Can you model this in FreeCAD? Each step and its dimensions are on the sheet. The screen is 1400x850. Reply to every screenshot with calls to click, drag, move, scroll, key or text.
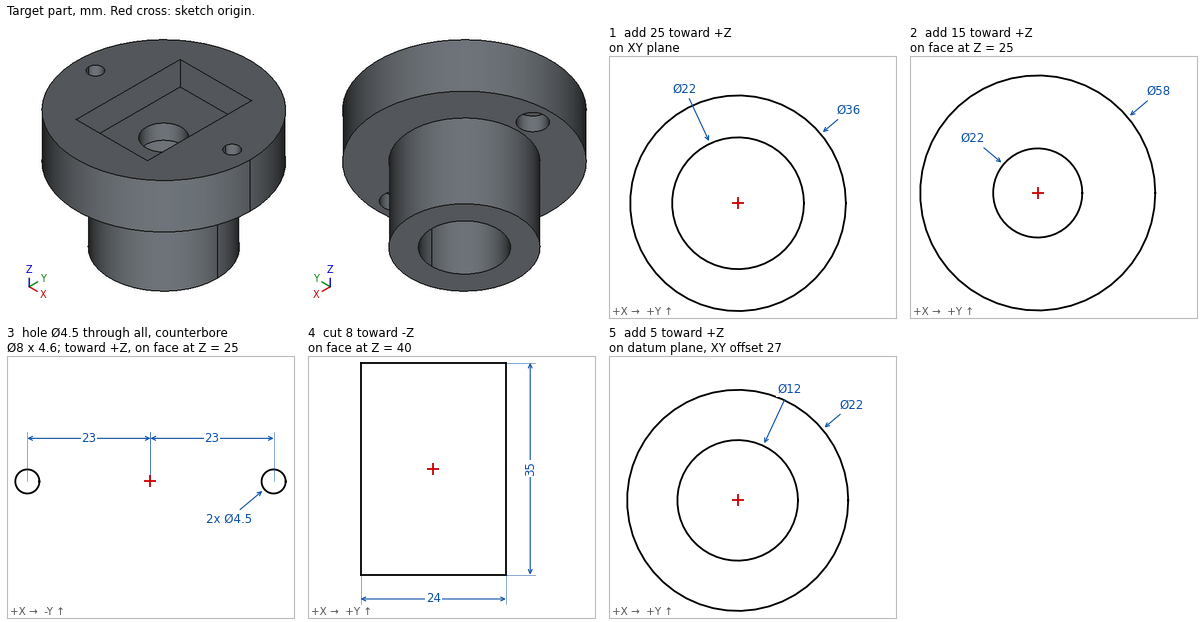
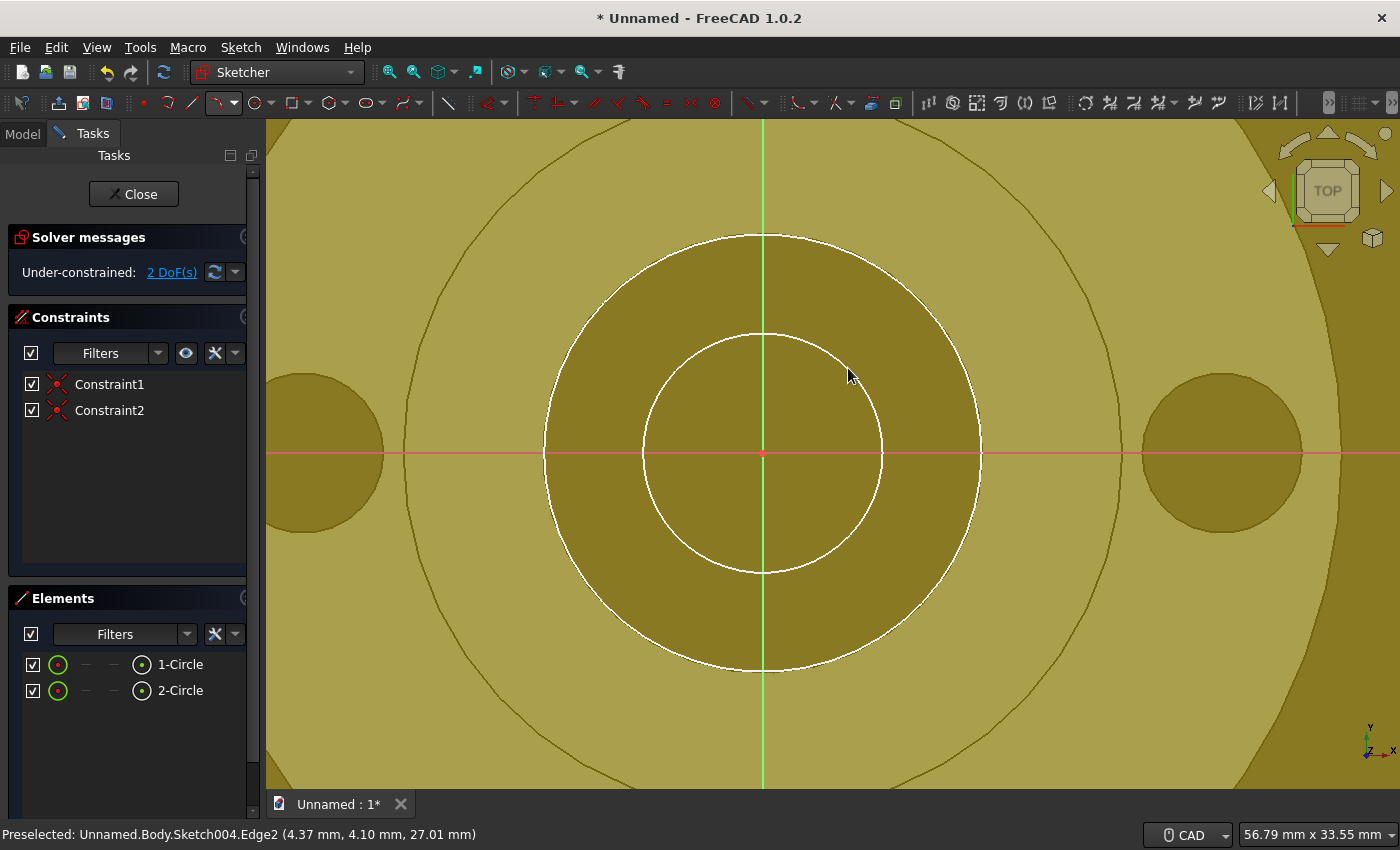
key(d)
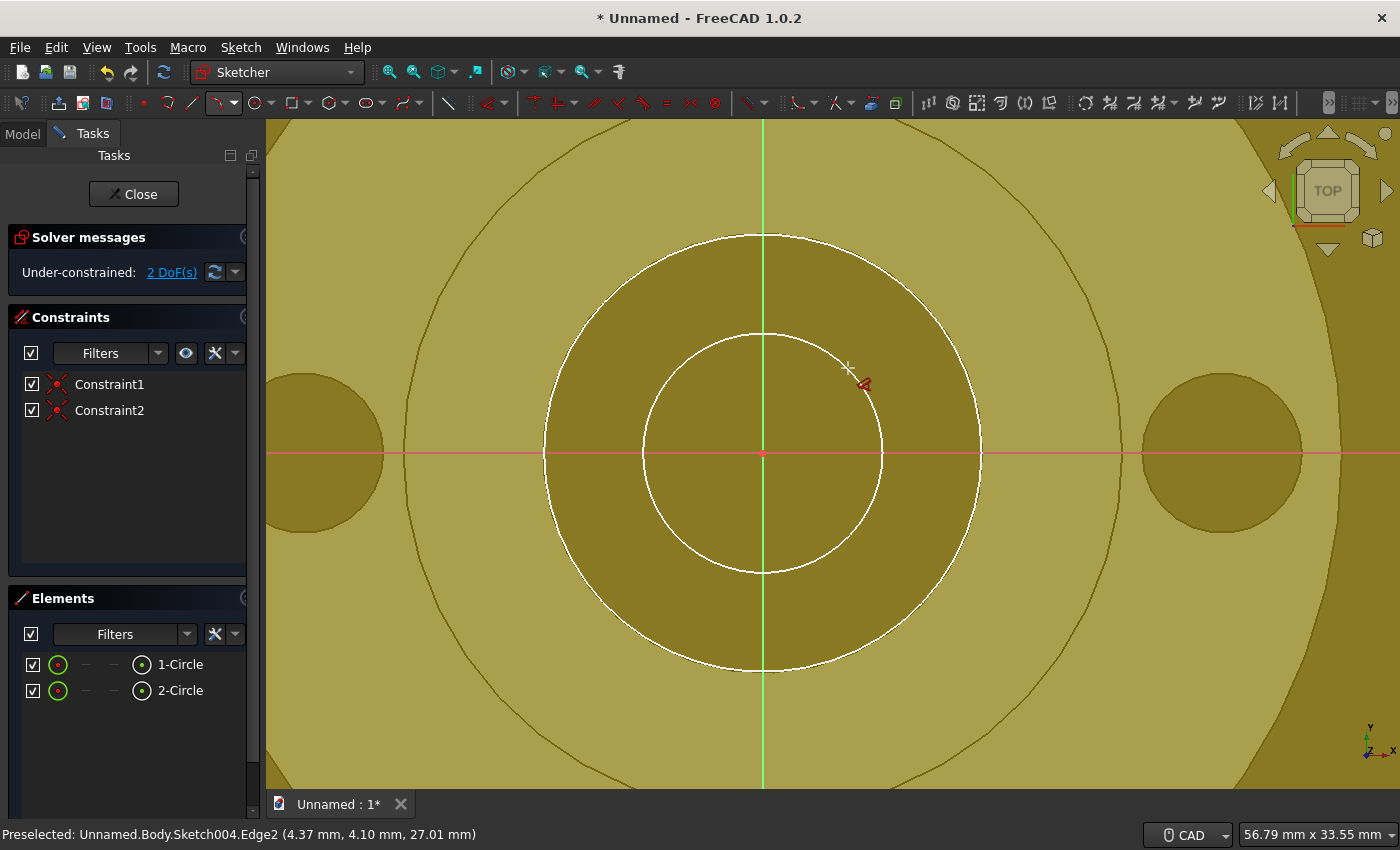
click(917, 298)
click(940, 275)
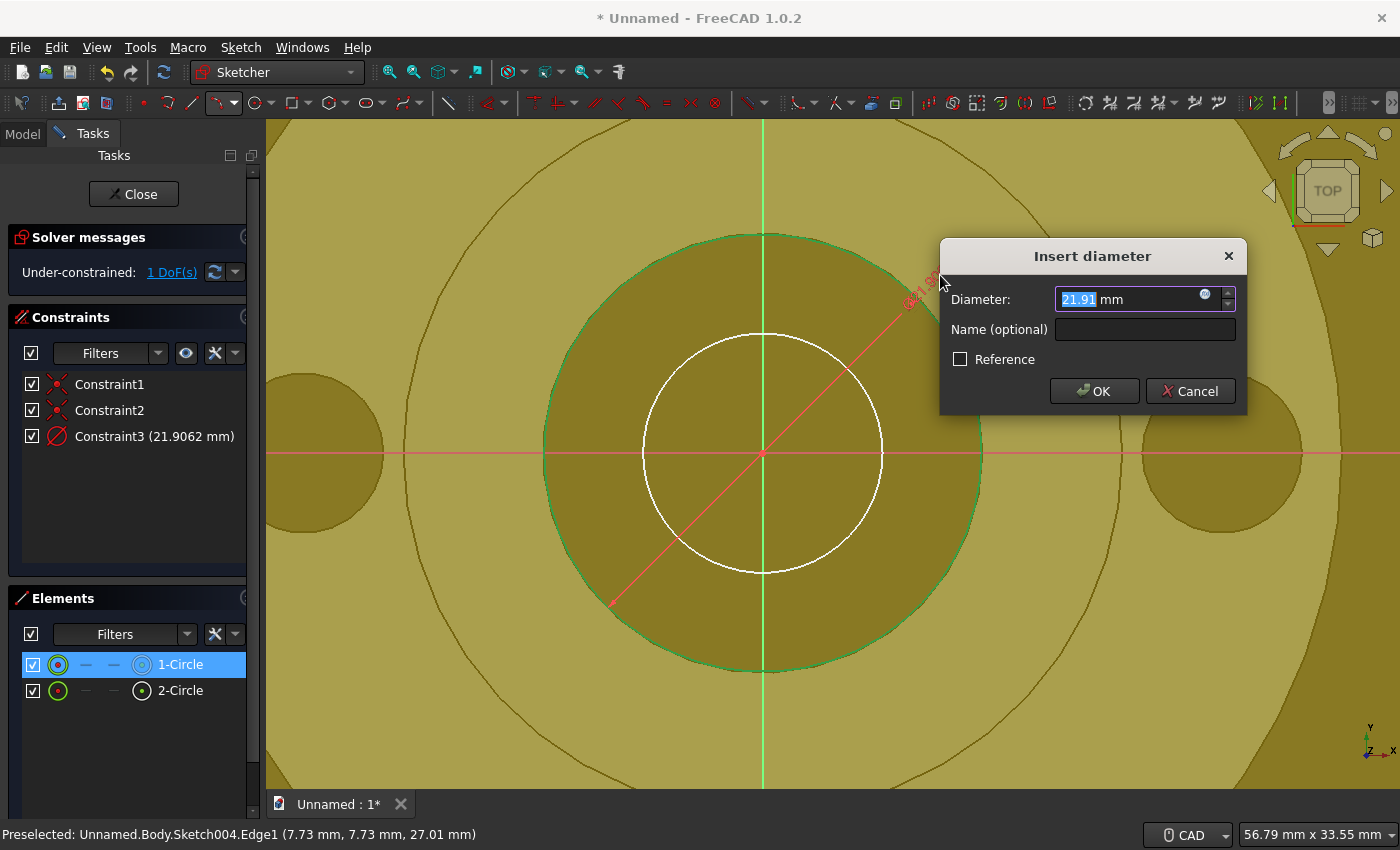
text(22)
key(Return)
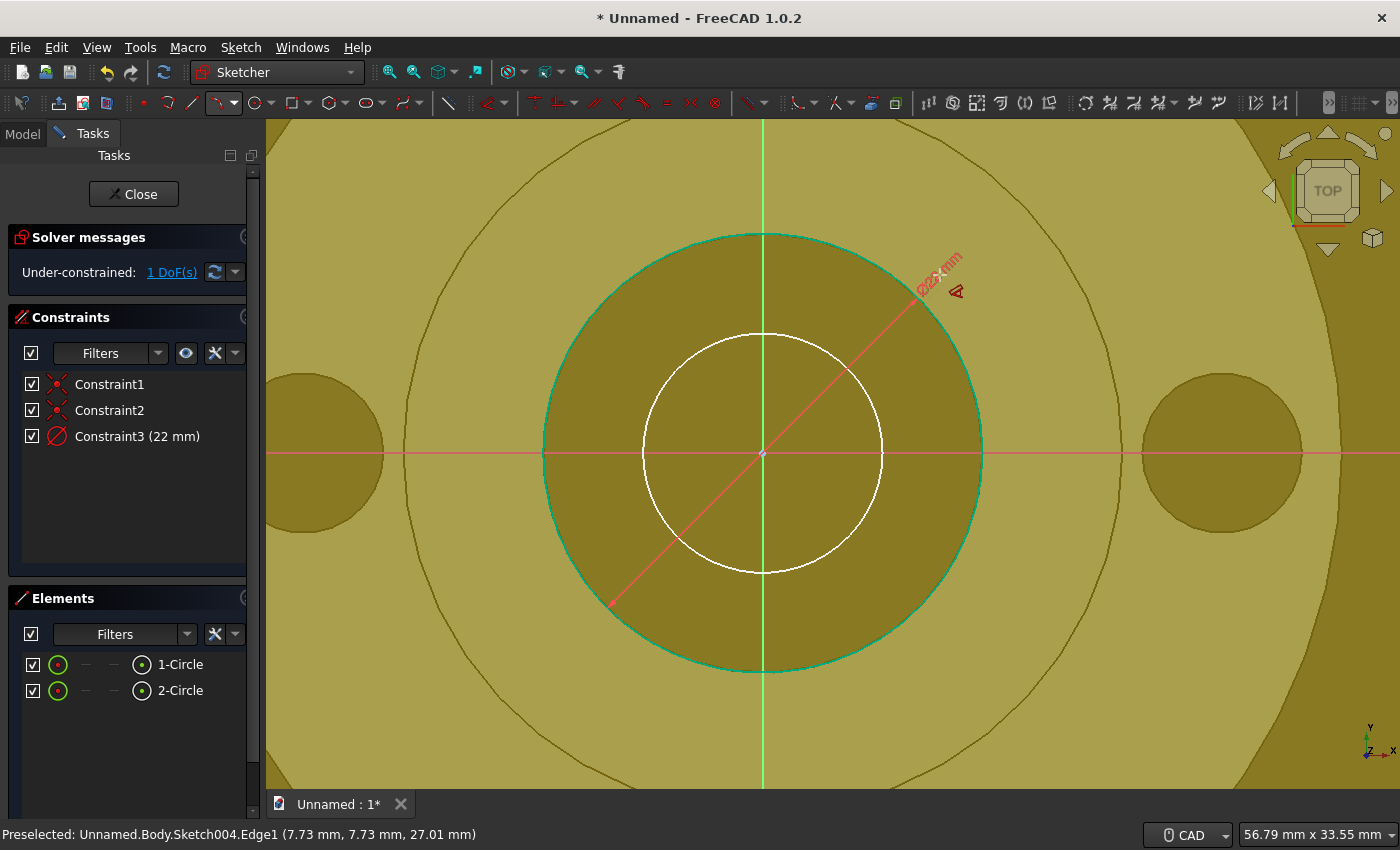
click(847, 368)
click(869, 345)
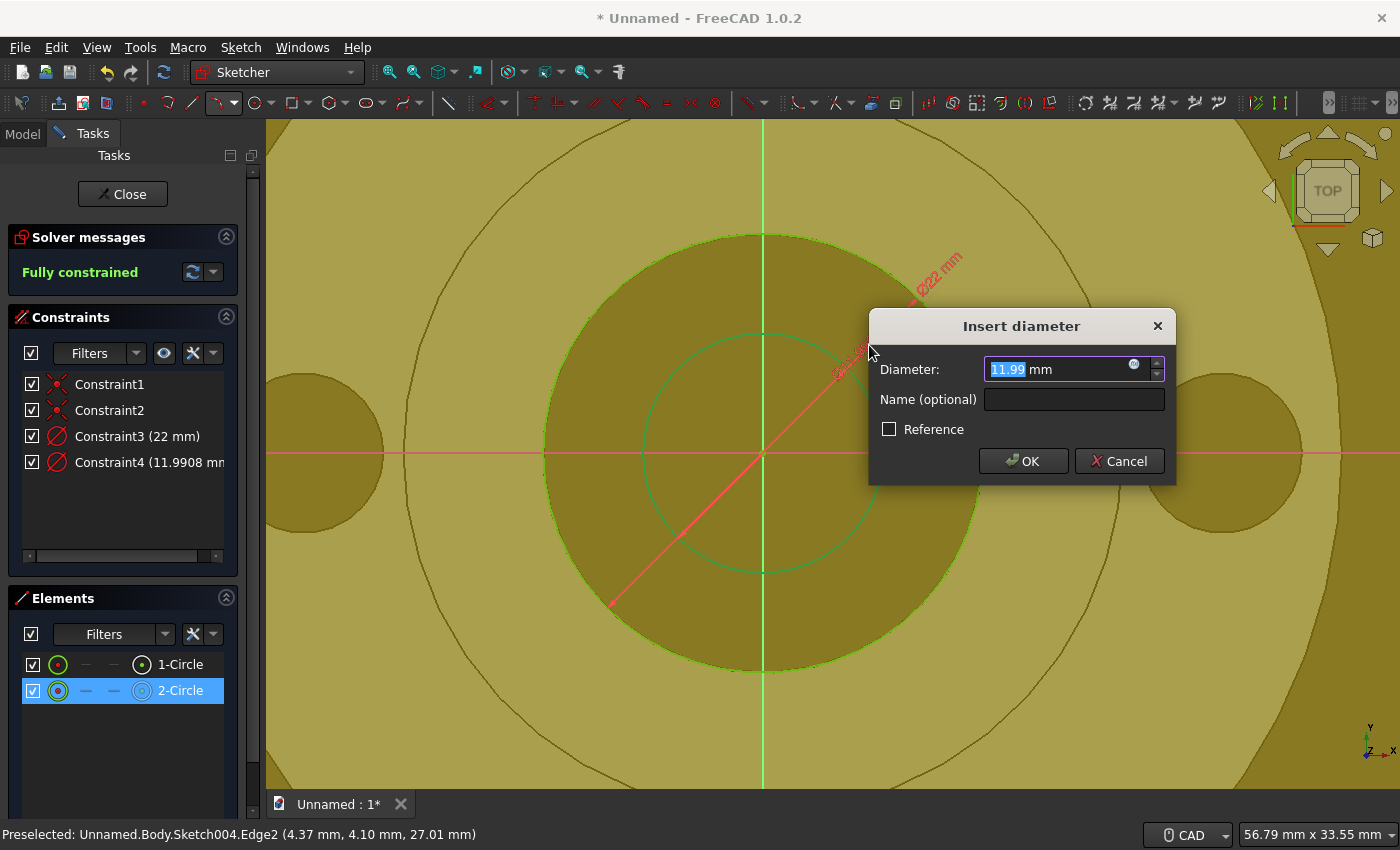
text(12)
key(Return)
key(Escape)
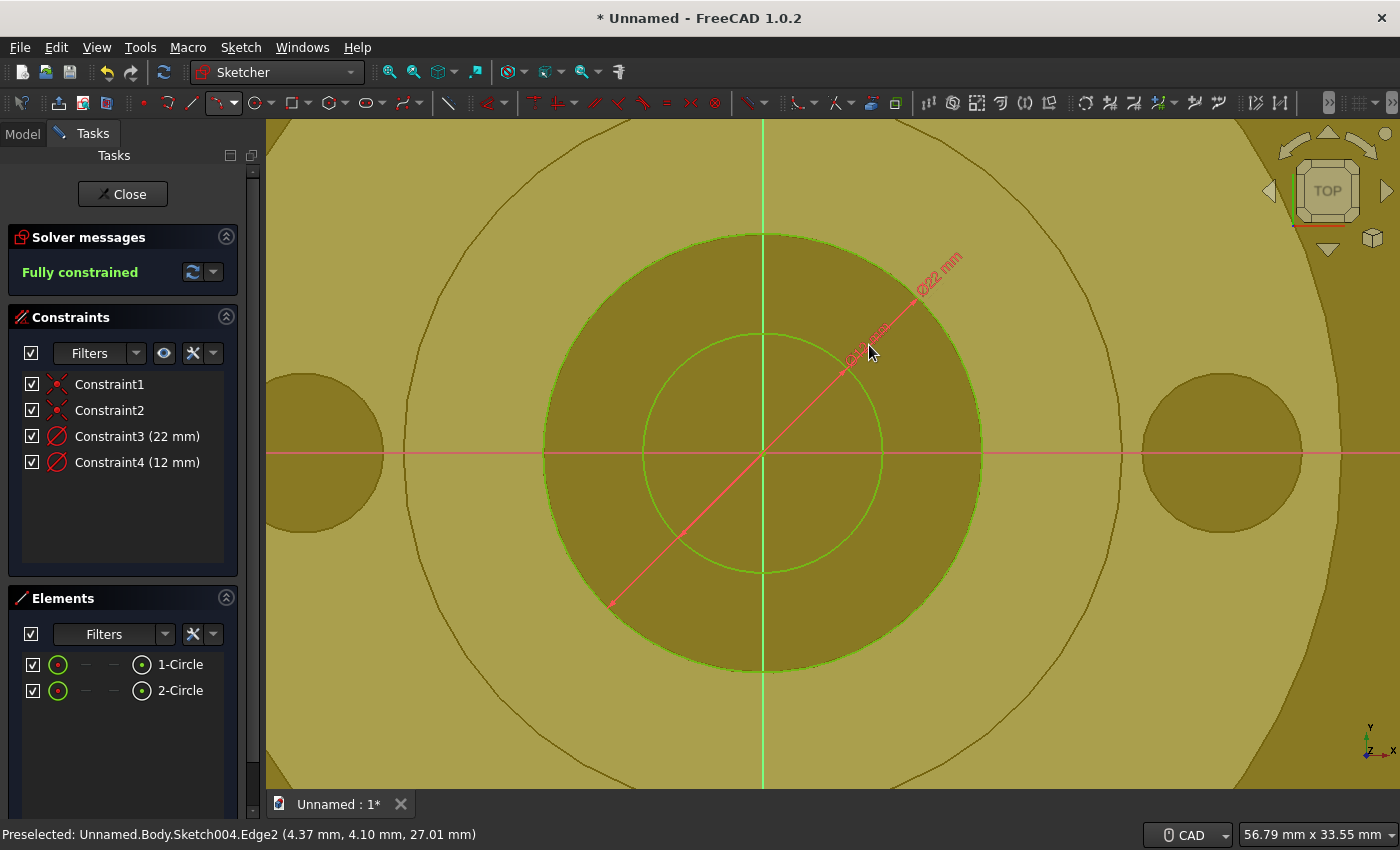
click(123, 194)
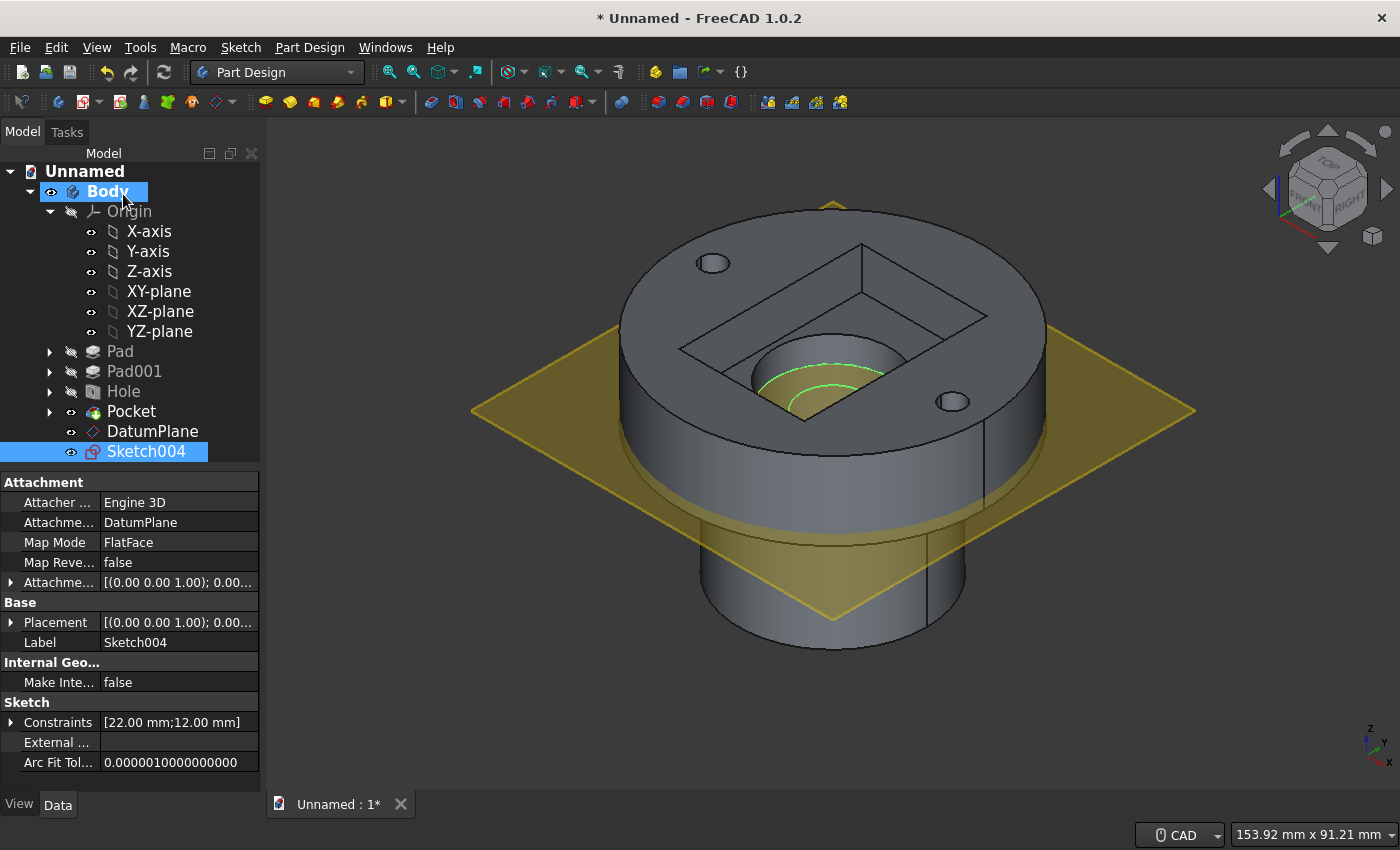
click(266, 102)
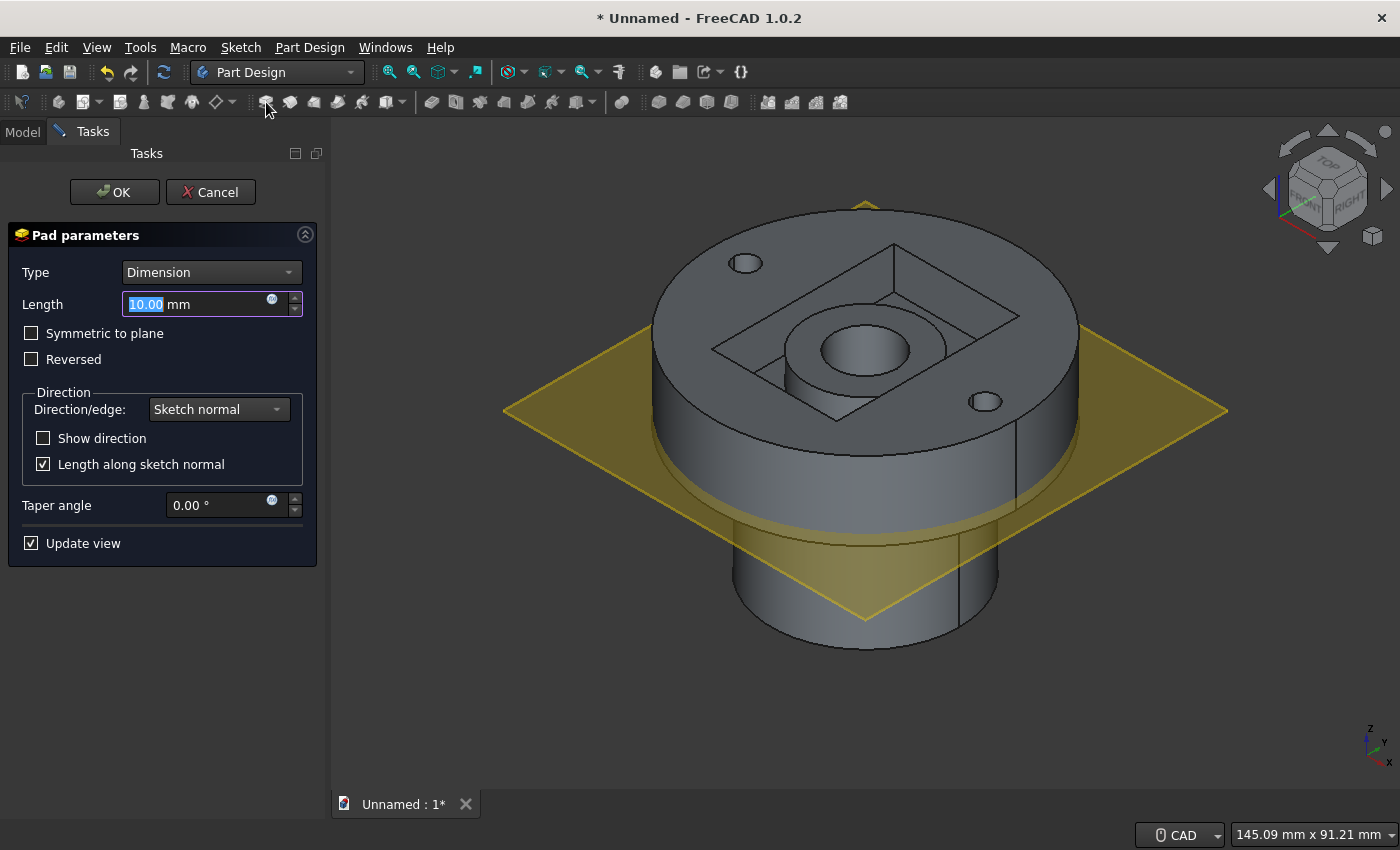
text(5)
key(Tab)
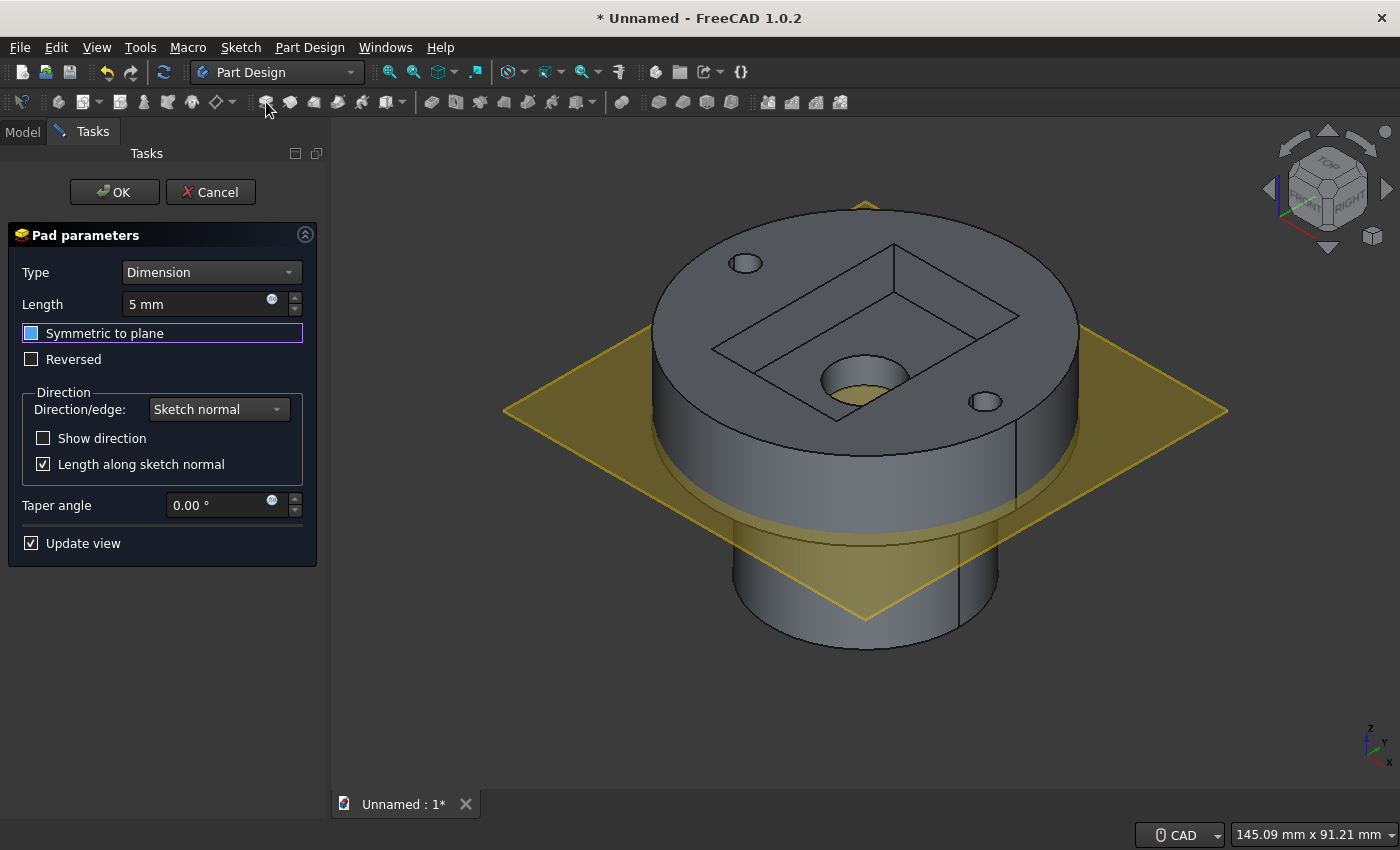
click(115, 192)